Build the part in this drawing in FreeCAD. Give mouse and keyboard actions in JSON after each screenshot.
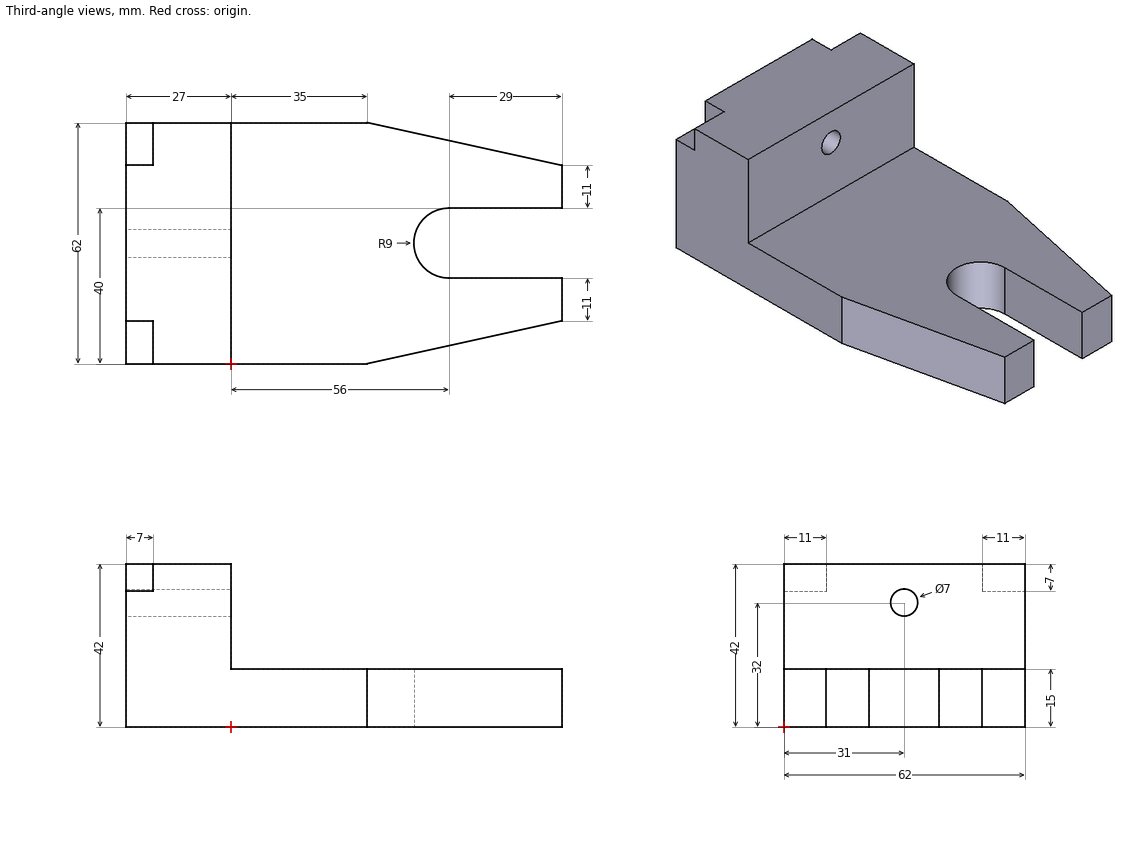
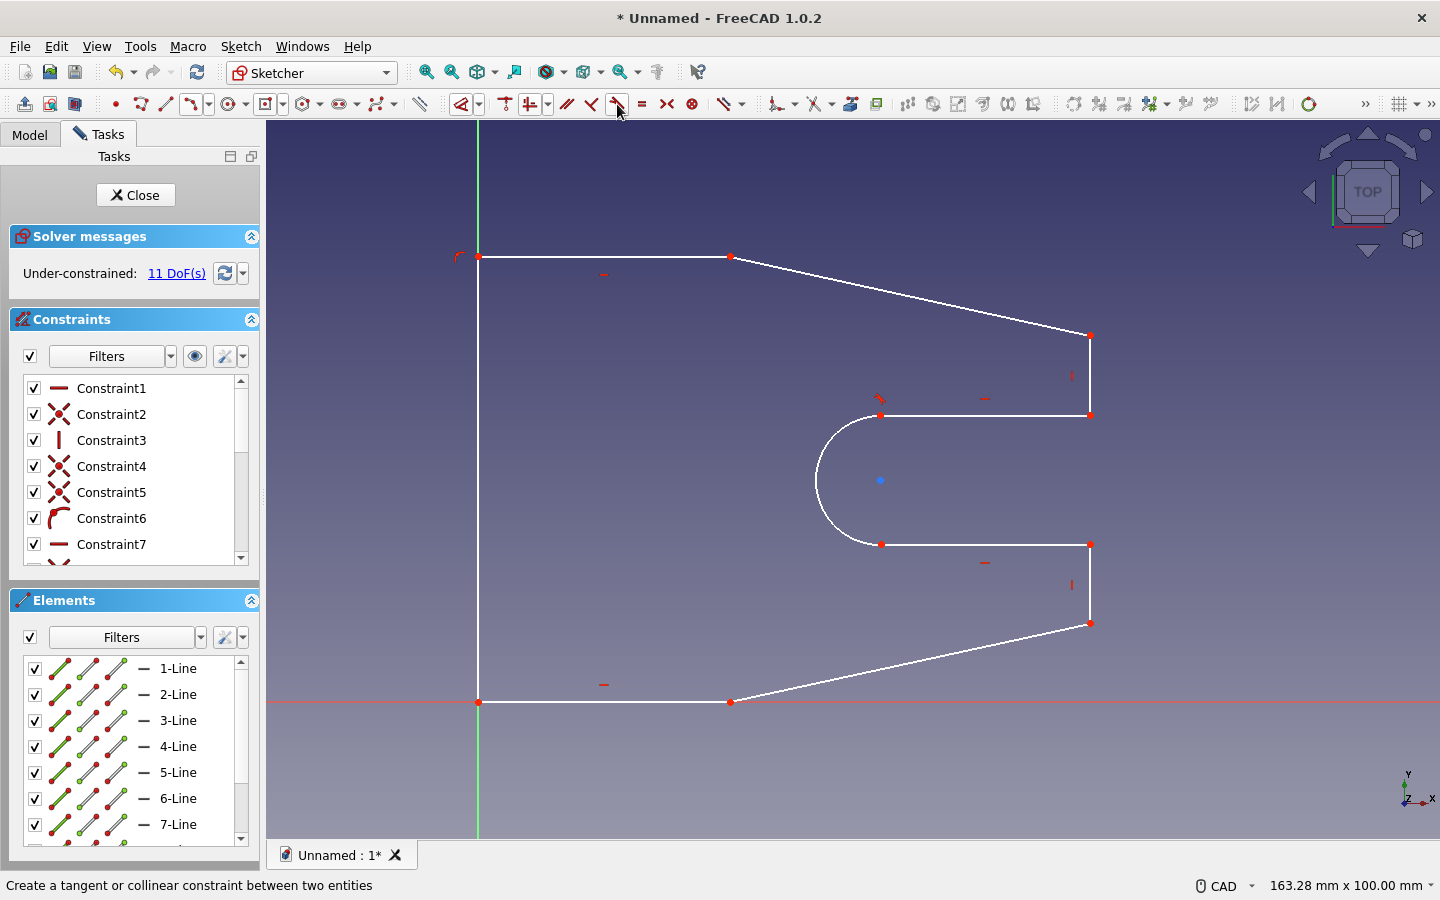
{"action": "left_click", "coordinate": [1027, 545]}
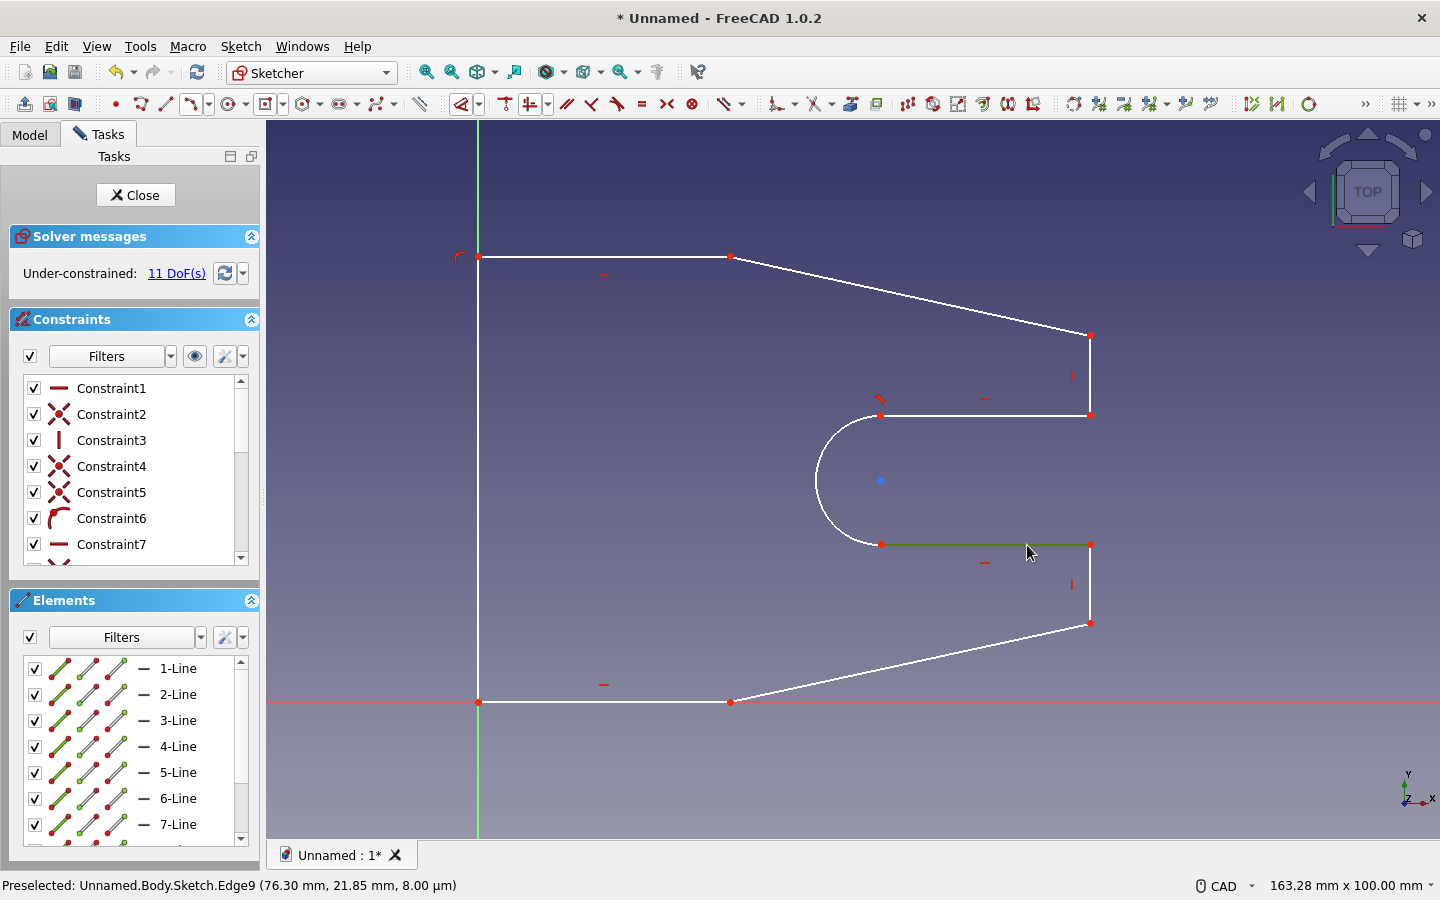
{"action": "left_click", "coordinate": [828, 443]}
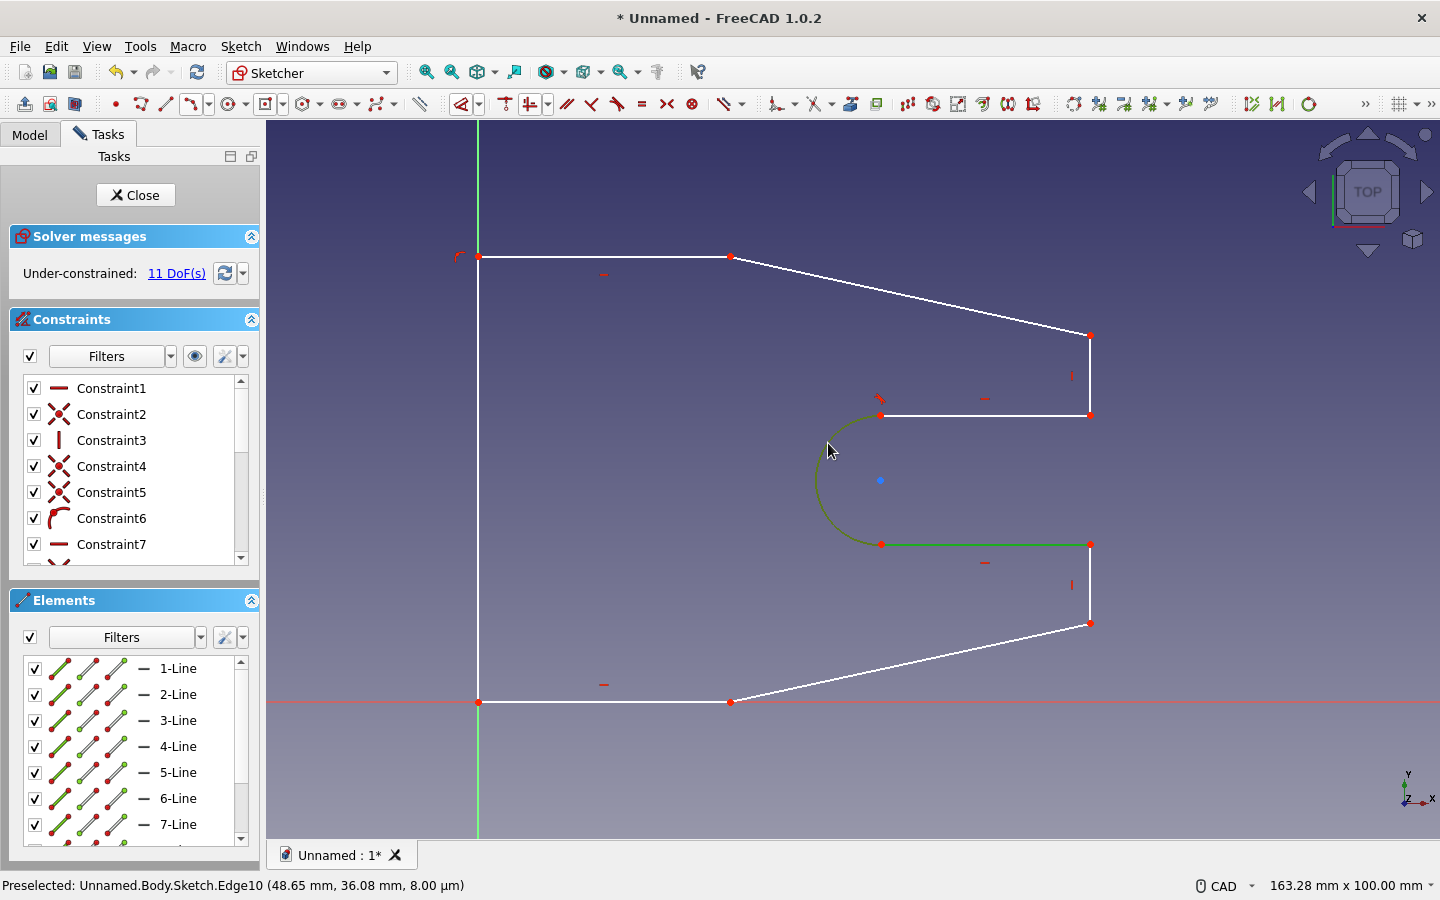
{"action": "left_click", "coordinate": [617, 104]}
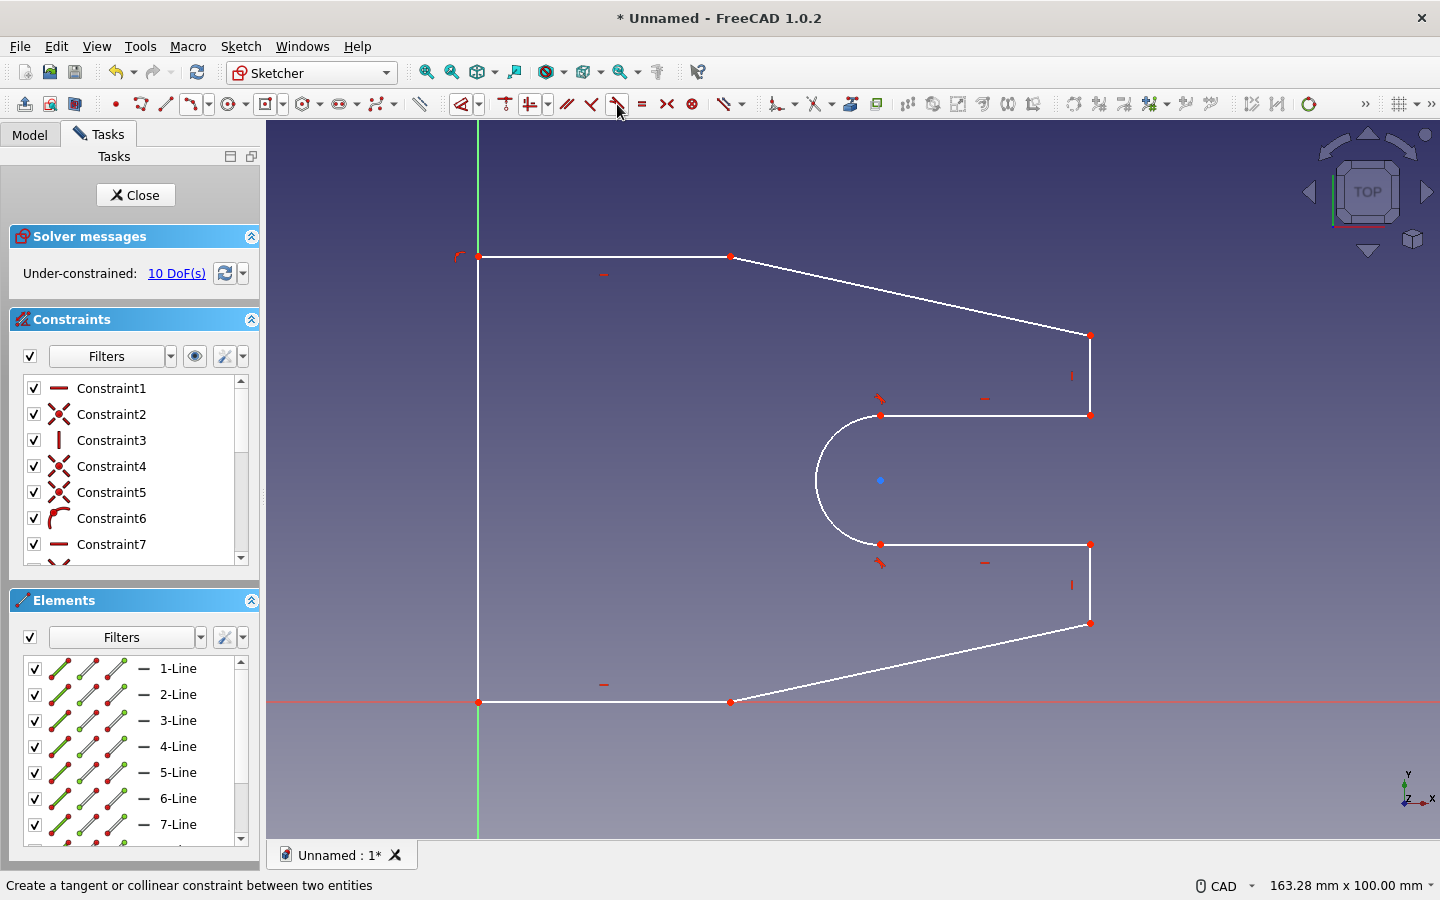
{"action": "left_click", "coordinate": [460, 104]}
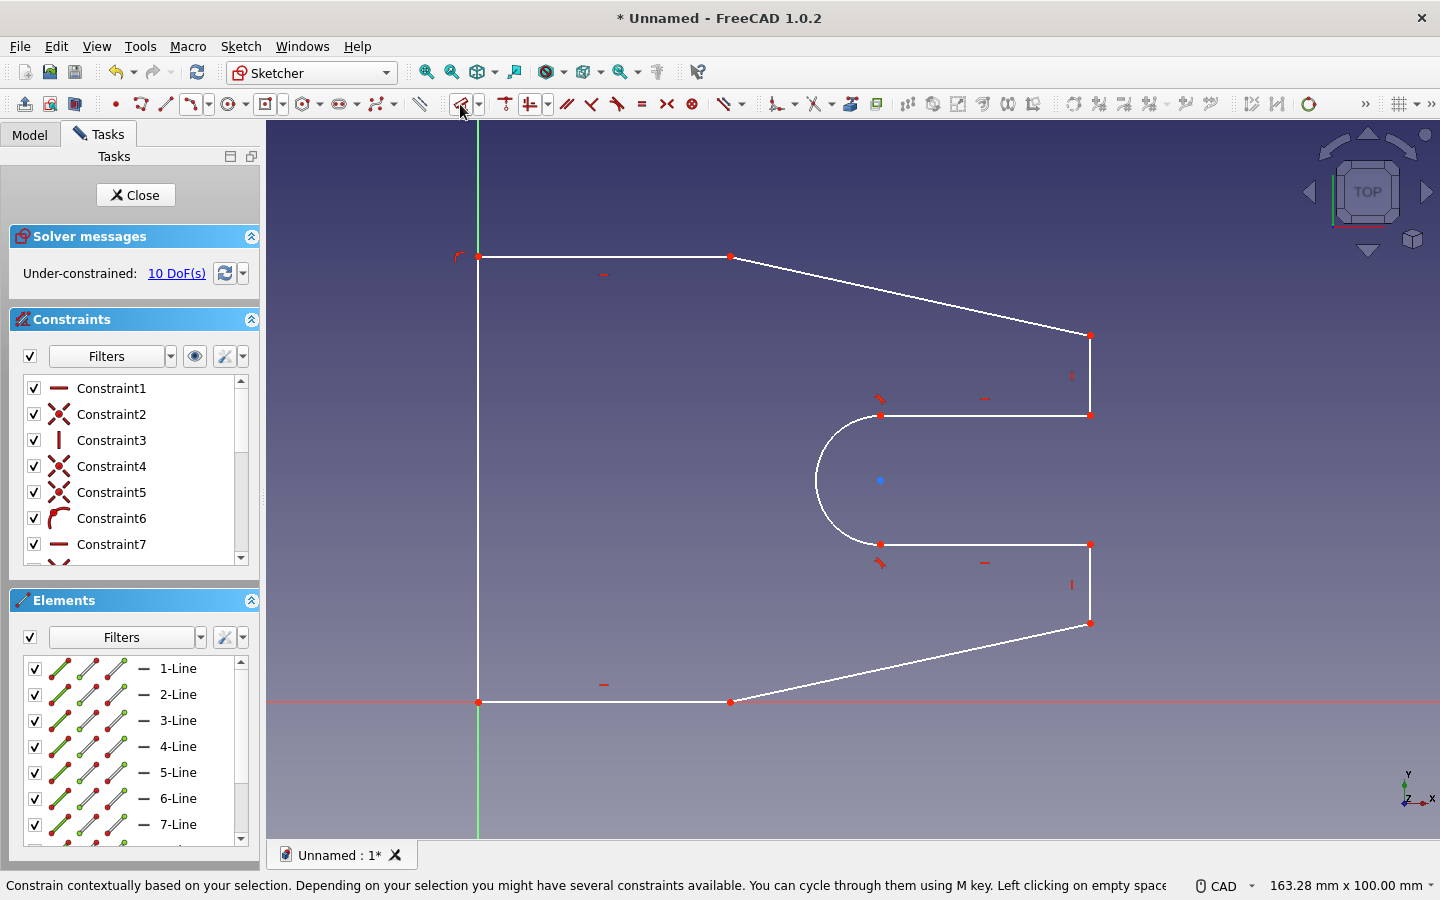
{"action": "left_click", "coordinate": [828, 443]}
{"action": "left_click", "coordinate": [802, 424]}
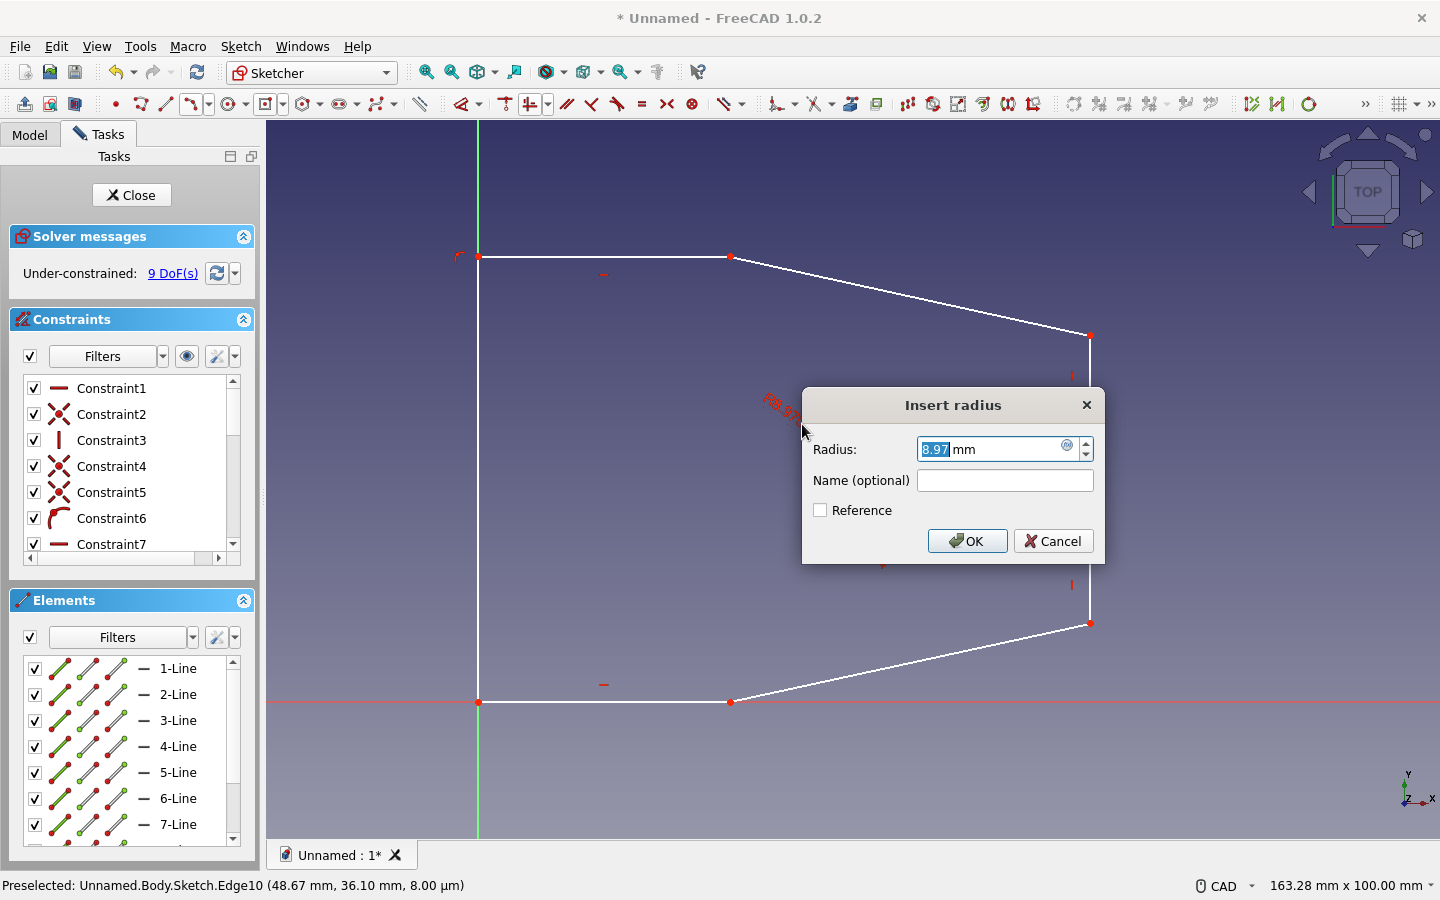
{"action": "type", "text": "9"}
{"action": "key", "text": "Return"}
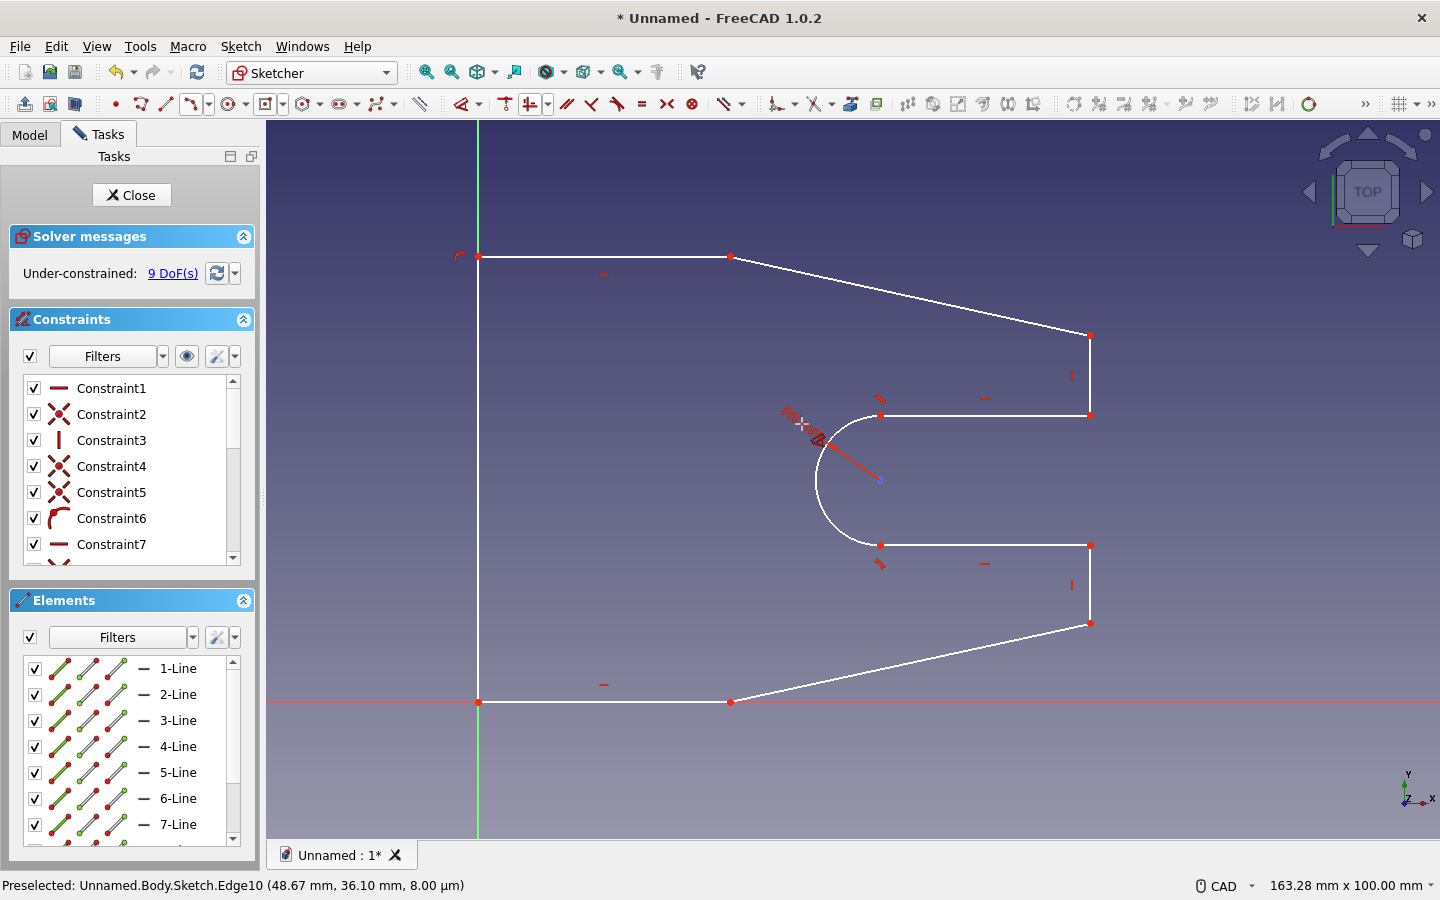
{"action": "left_click", "coordinate": [943, 416]}
{"action": "left_click", "coordinate": [985, 382]}